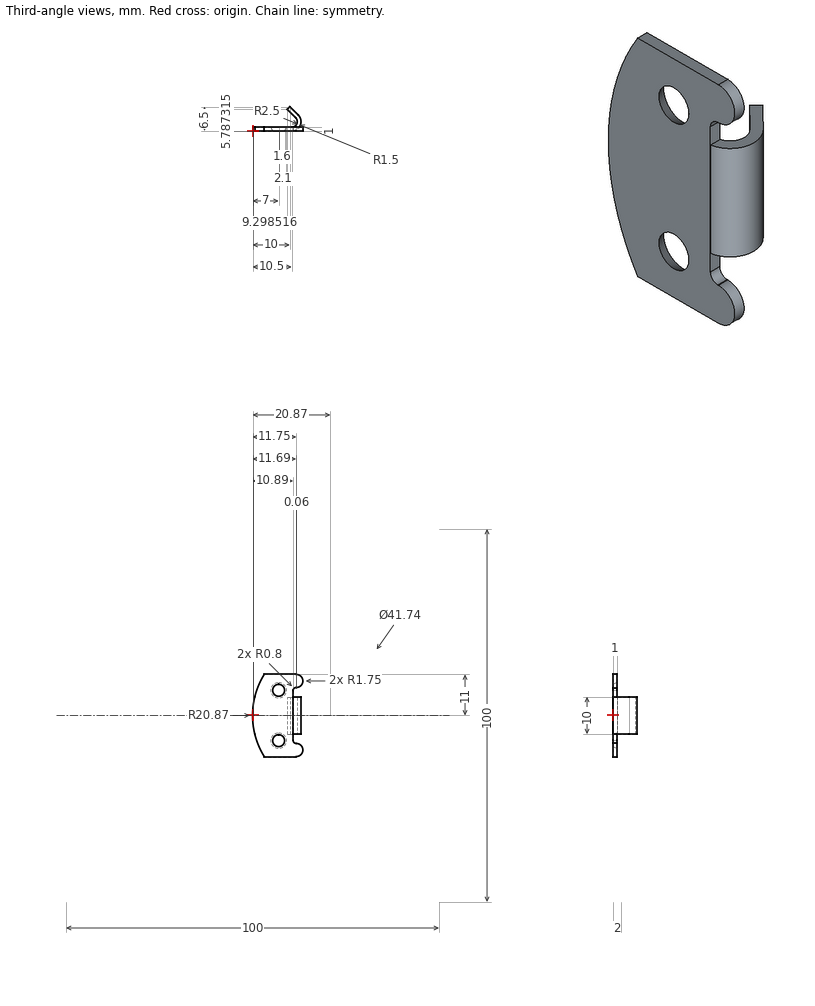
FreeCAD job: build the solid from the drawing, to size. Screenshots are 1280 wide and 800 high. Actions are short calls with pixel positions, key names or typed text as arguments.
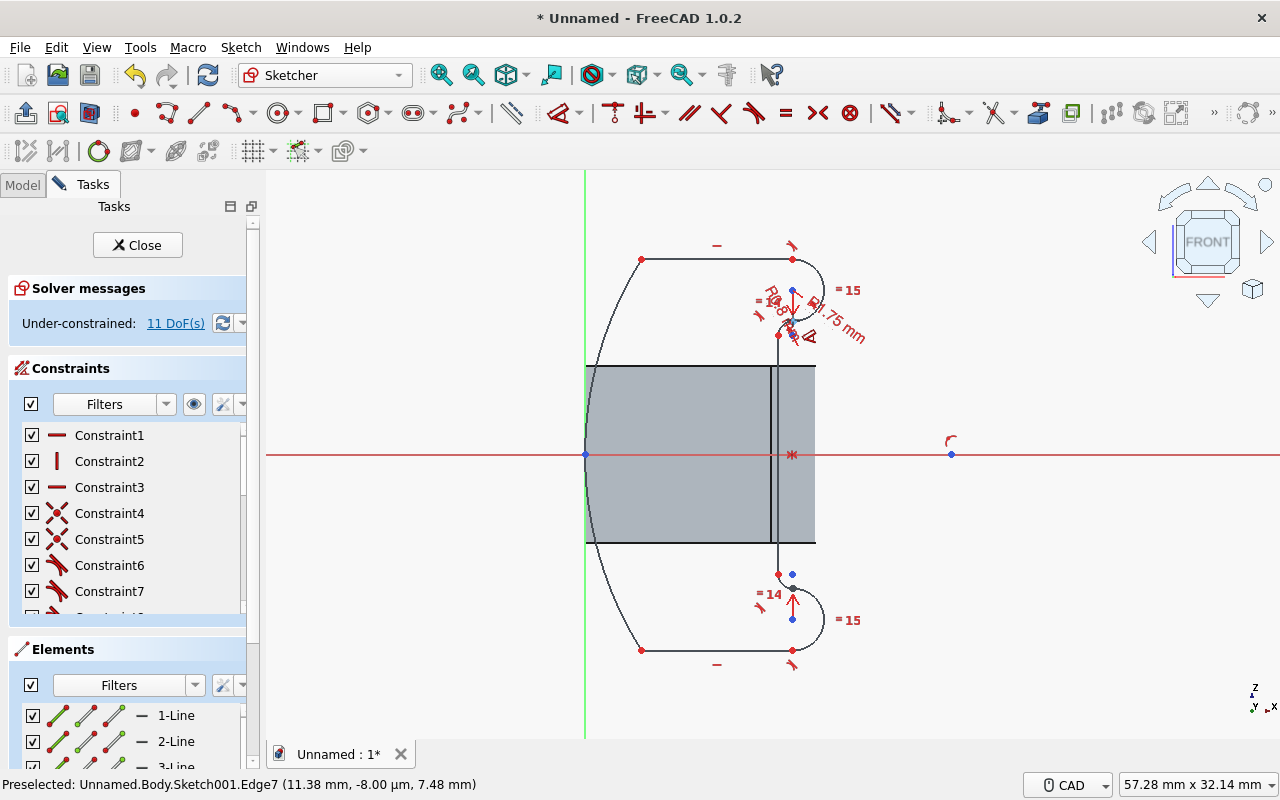
scroll(594, 373, up, 3)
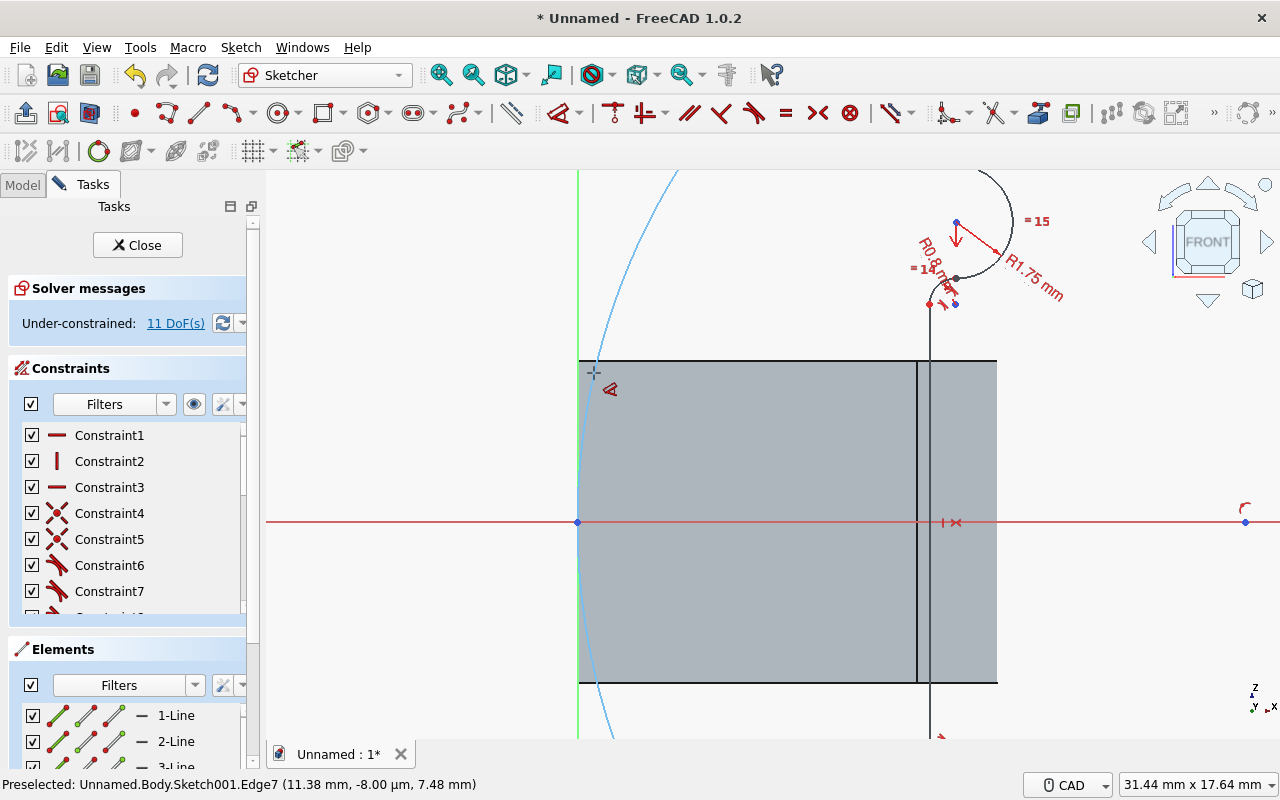
click(594, 373)
click(563, 366)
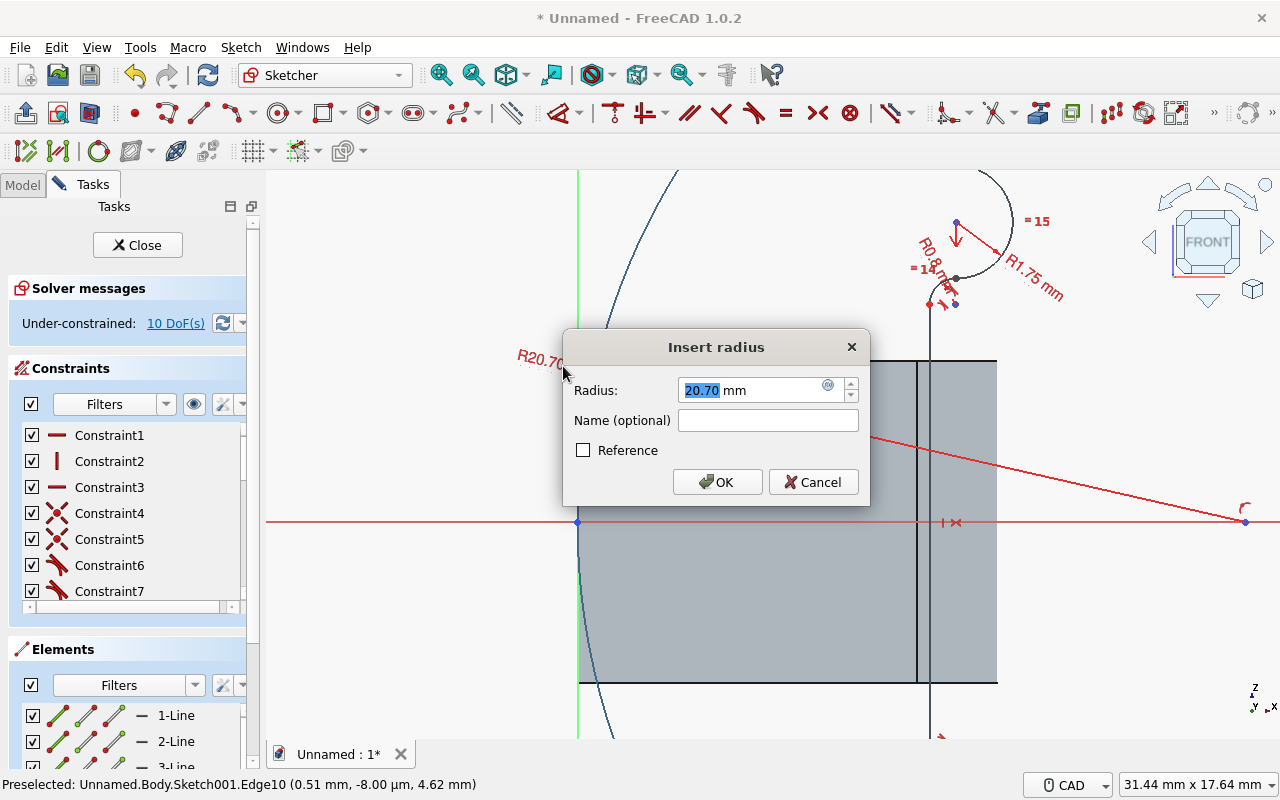
text(20.87)
key(Return)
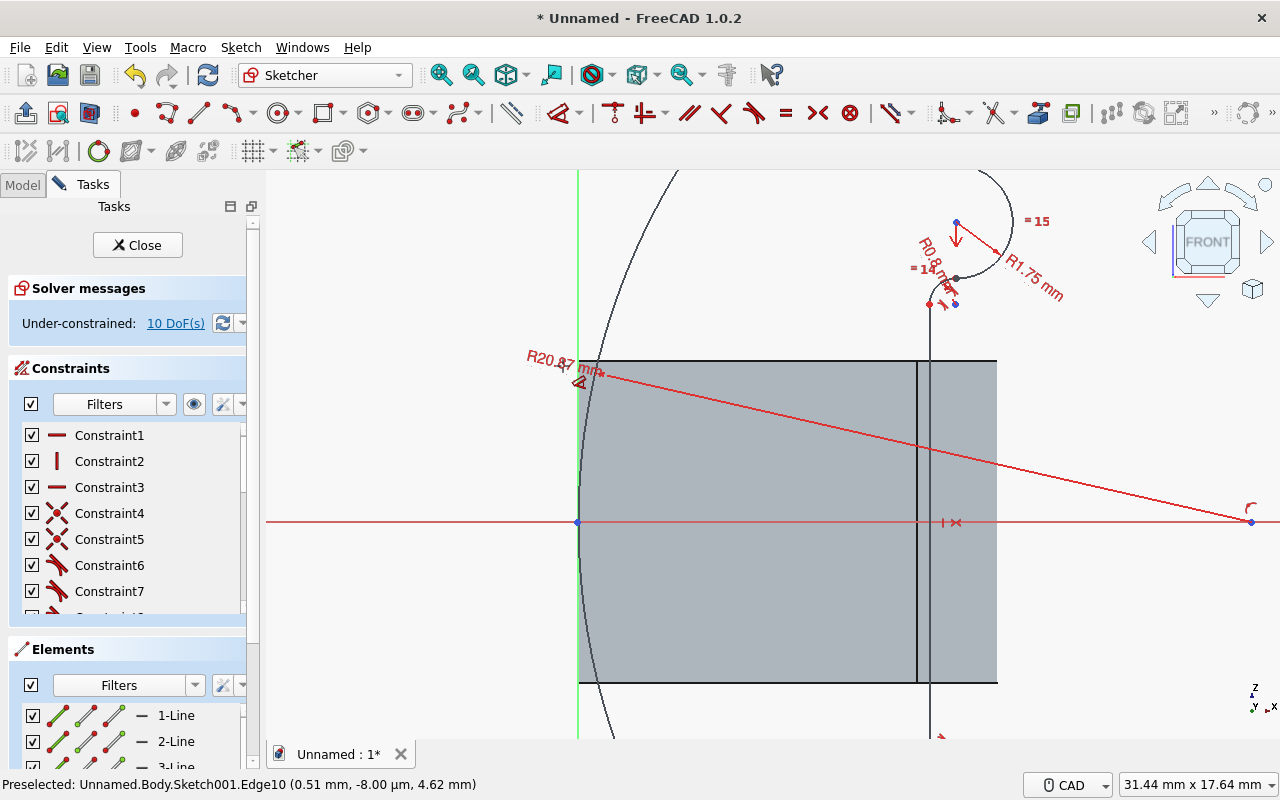
scroll(594, 372, down, 3)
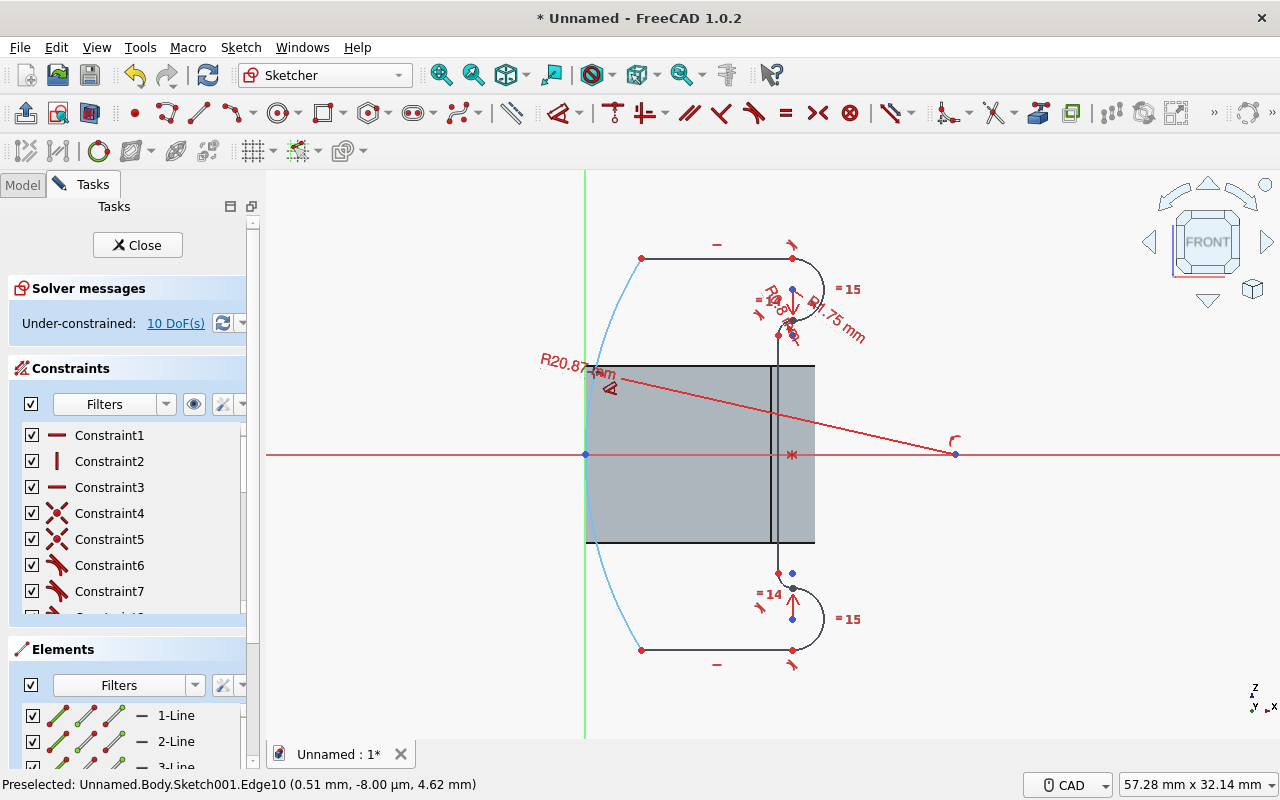
click(642, 259)
click(551, 312)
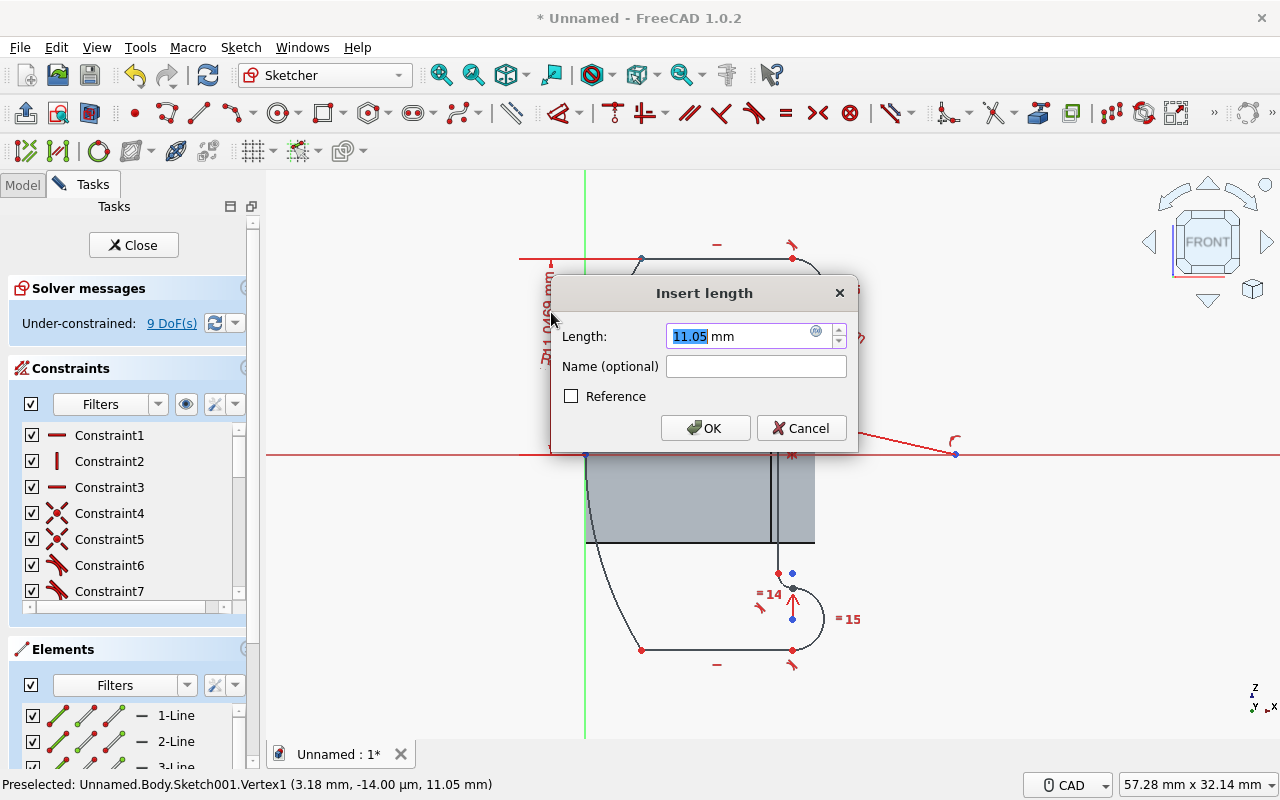
text(11)
key(Return)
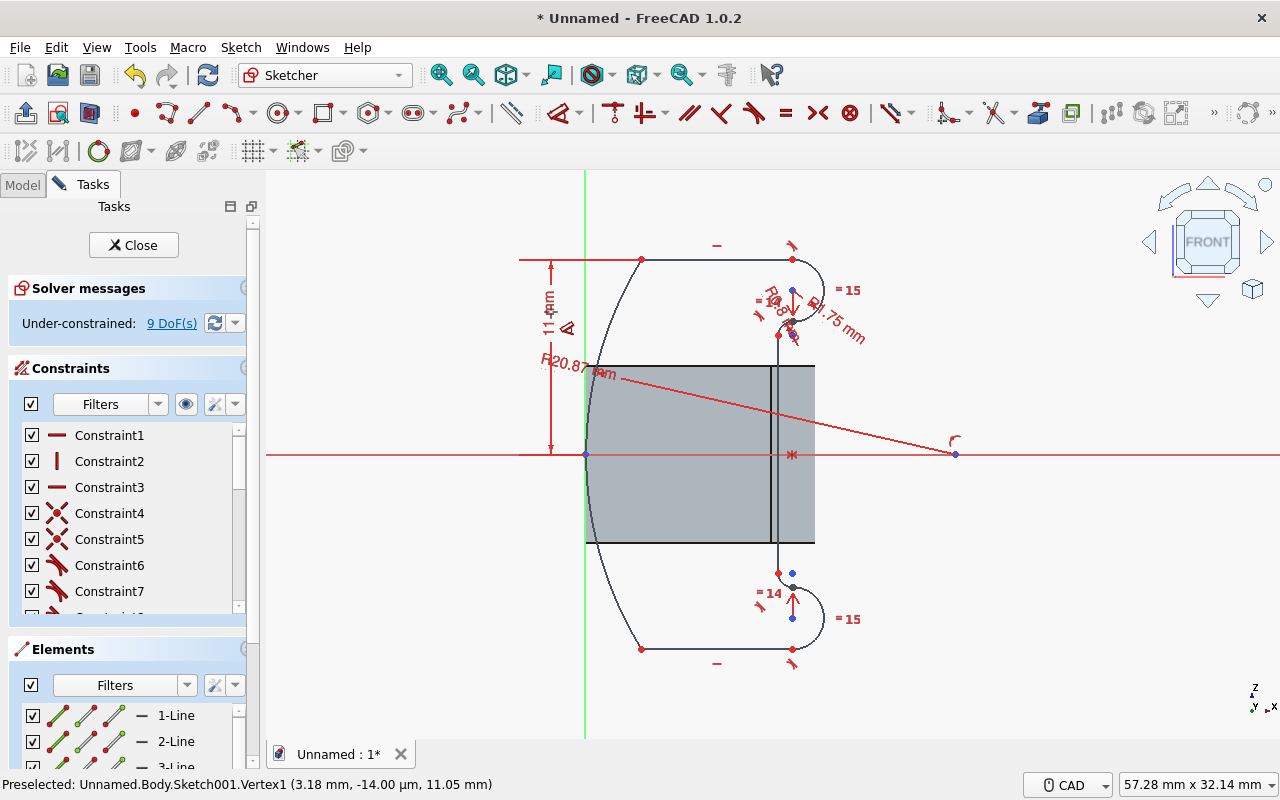
scroll(793, 322, up, 19)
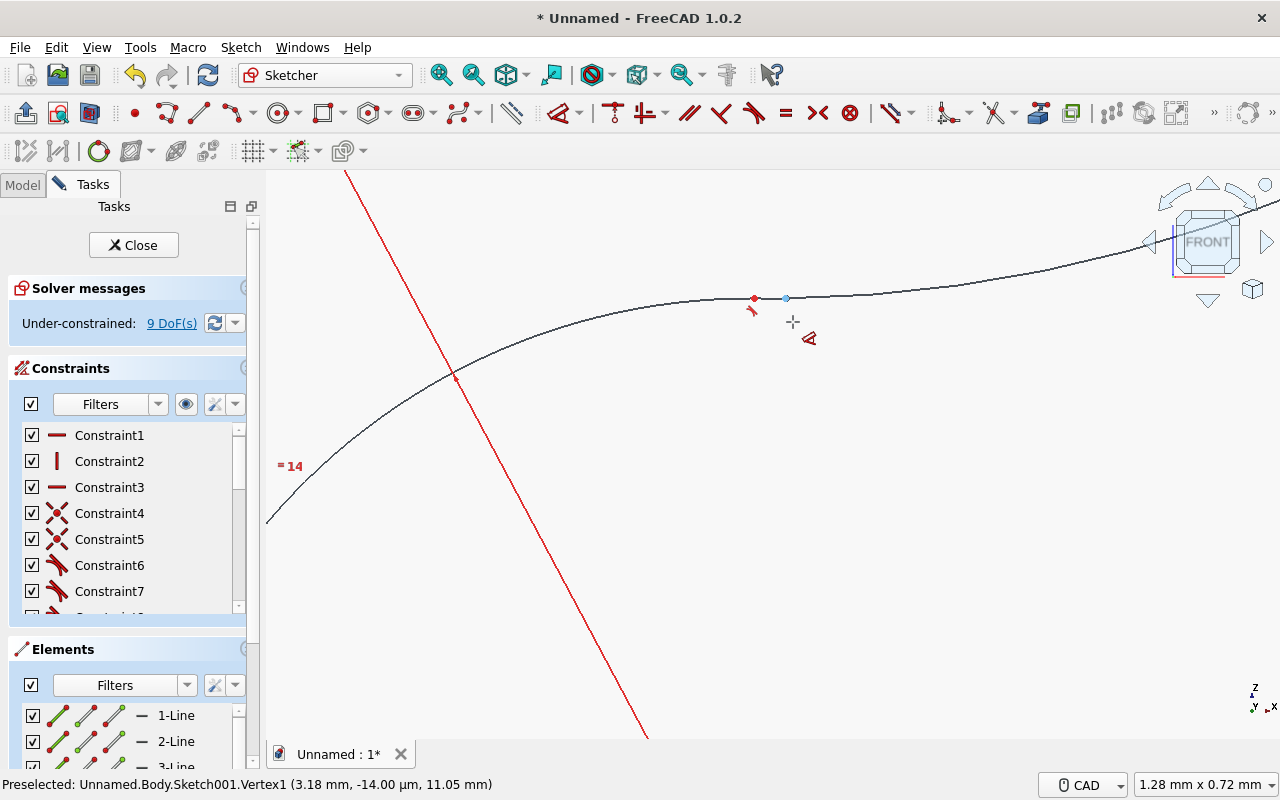
click(770, 299)
click(770, 264)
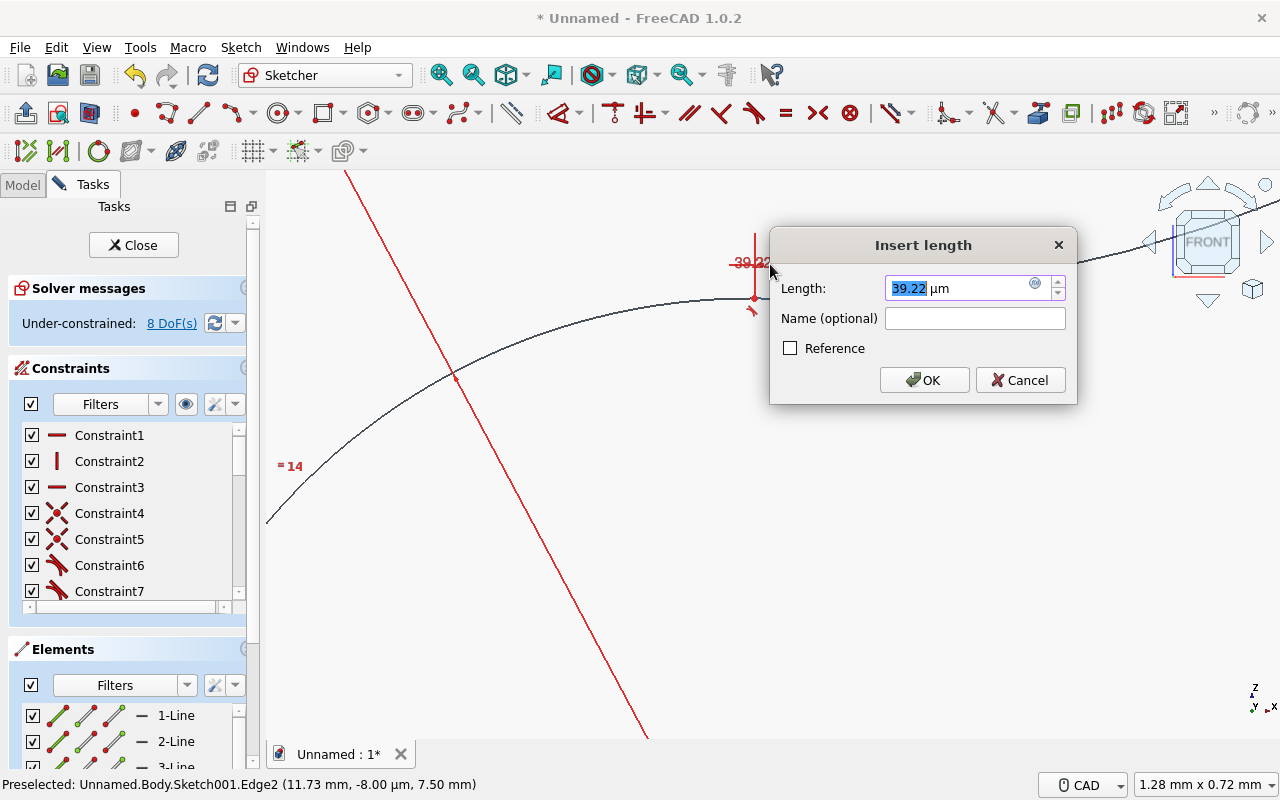
key(ctrl+a)
text(0.06 mm)
key(Return)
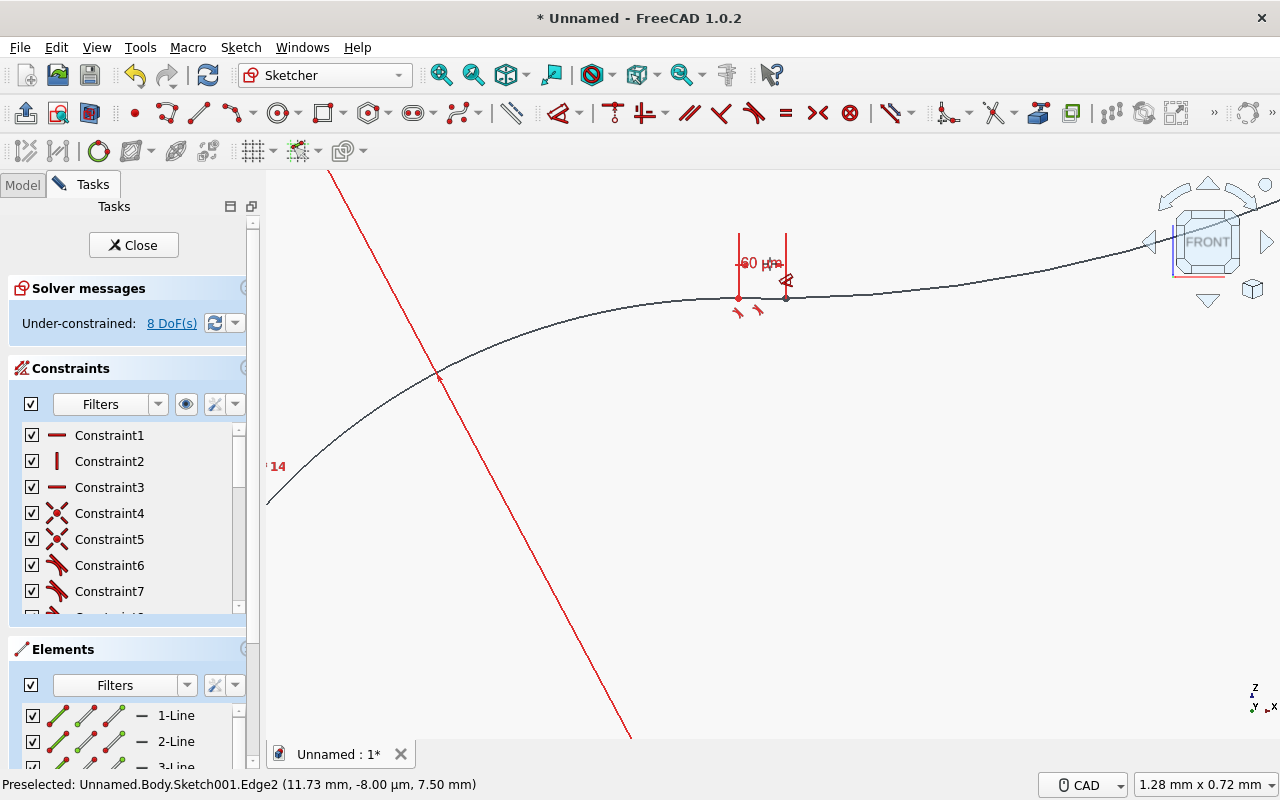
scroll(704, 454, down, 15)